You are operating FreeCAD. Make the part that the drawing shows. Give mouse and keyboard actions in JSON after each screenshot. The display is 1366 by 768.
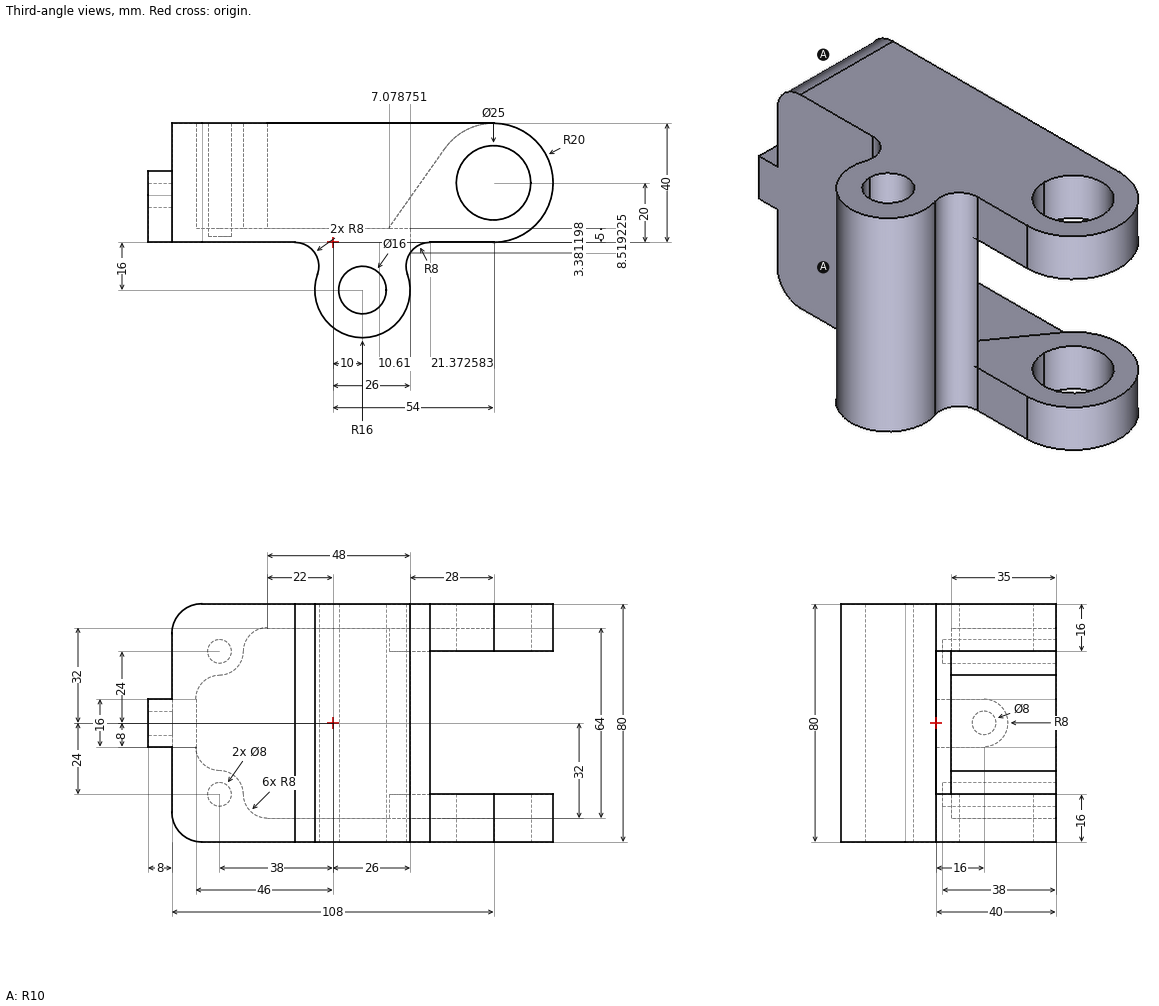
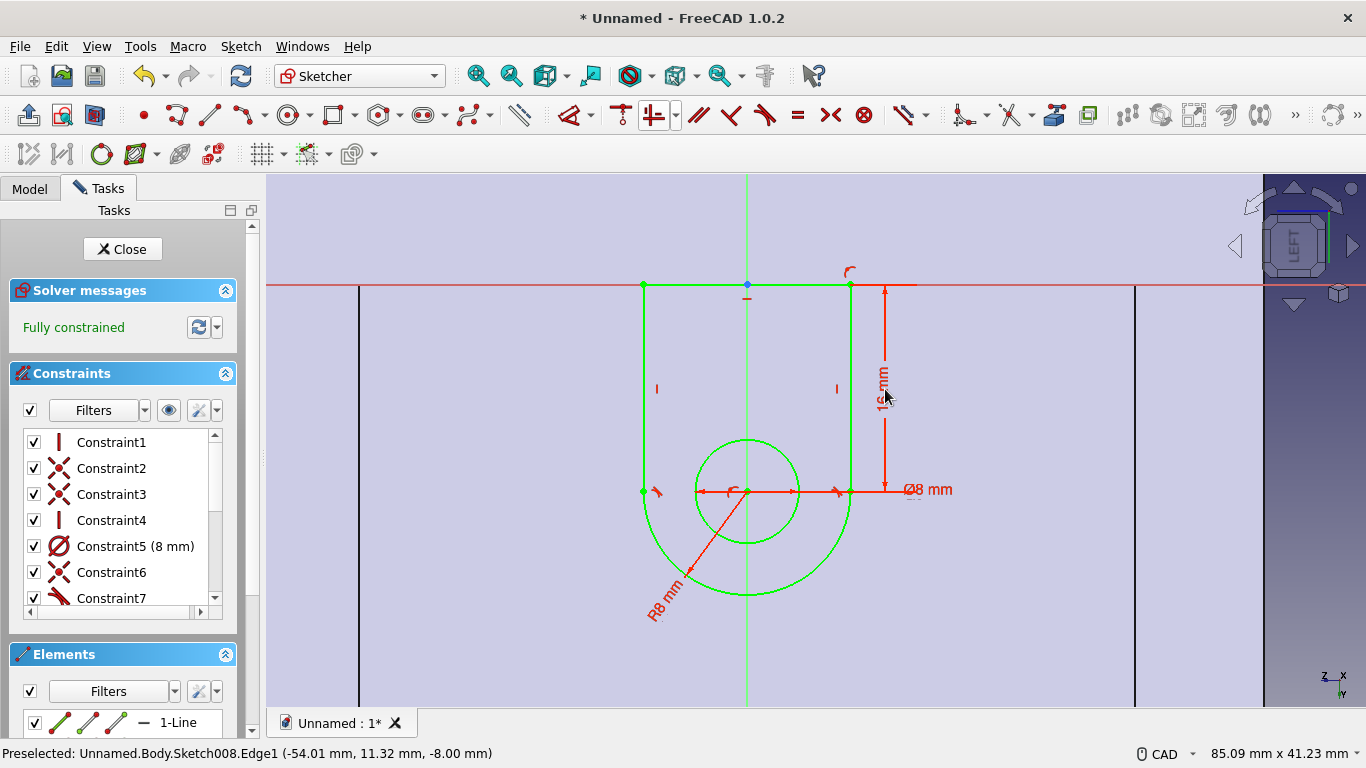
{"action": "left_click", "coordinate": [123, 249]}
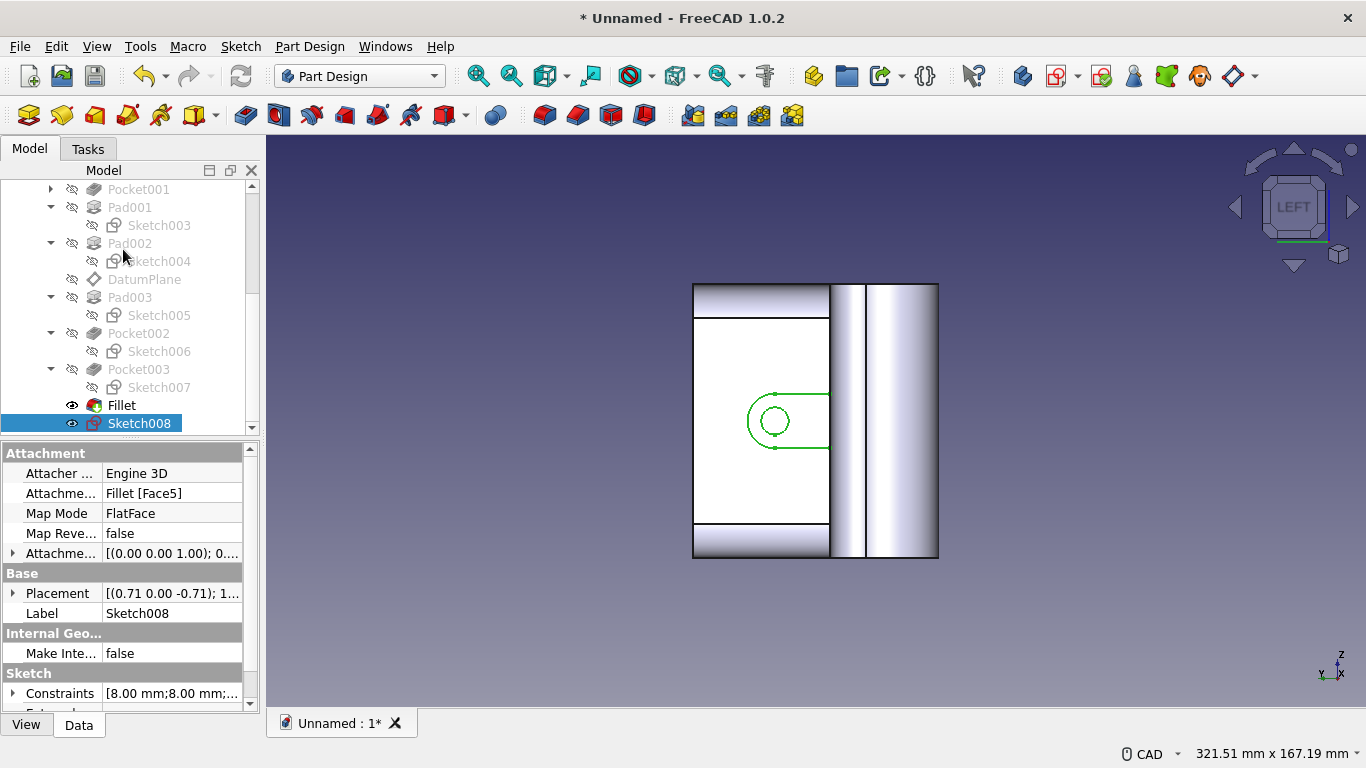
{"action": "left_click", "coordinate": [29, 116]}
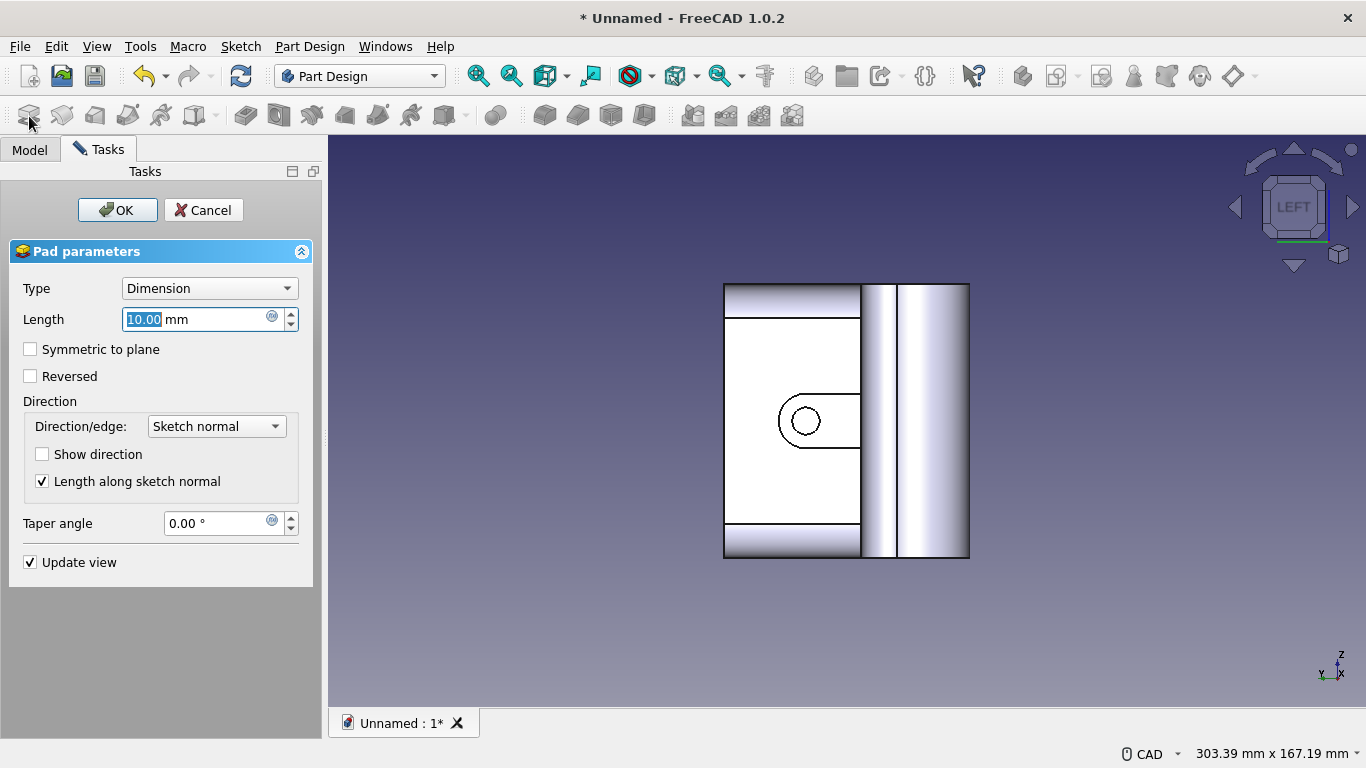
{"action": "type", "text": "8"}
{"action": "key", "text": "Tab"}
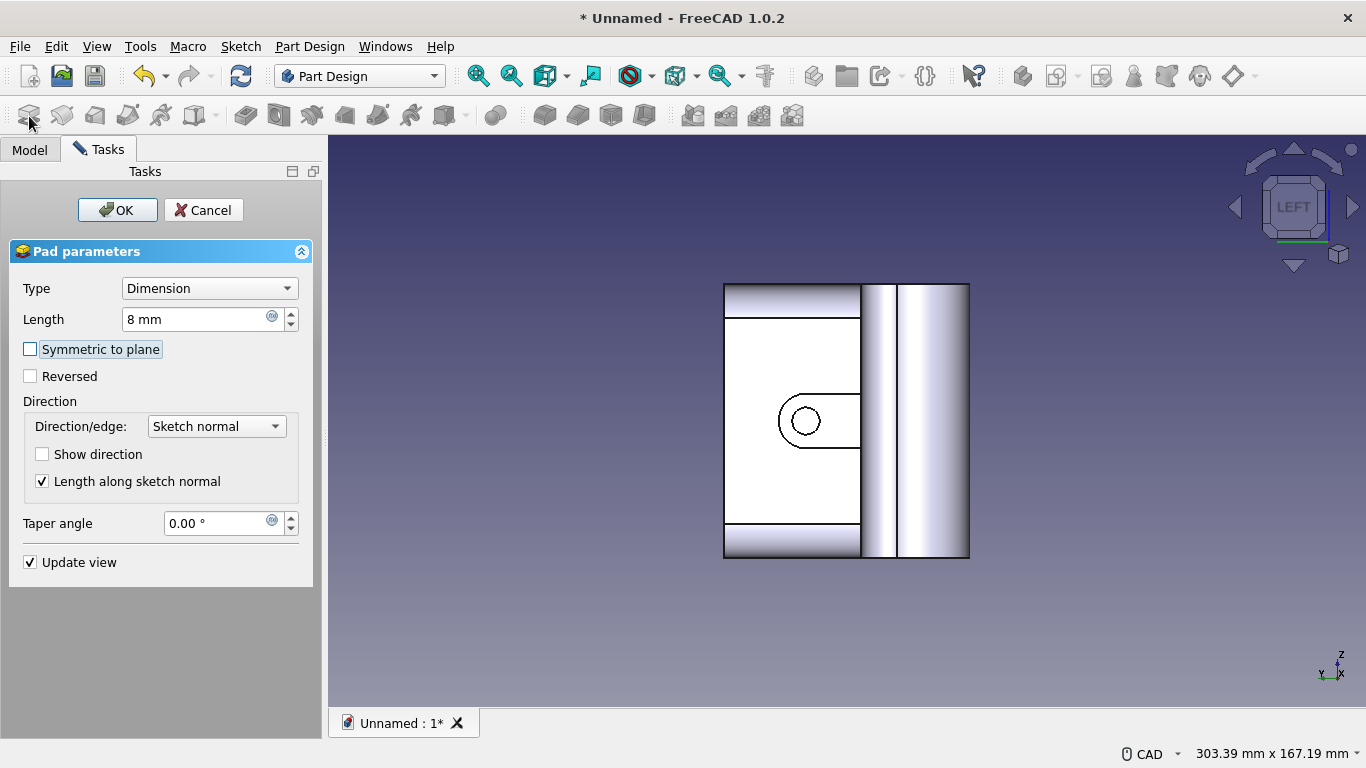
{"action": "left_click", "coordinate": [118, 210]}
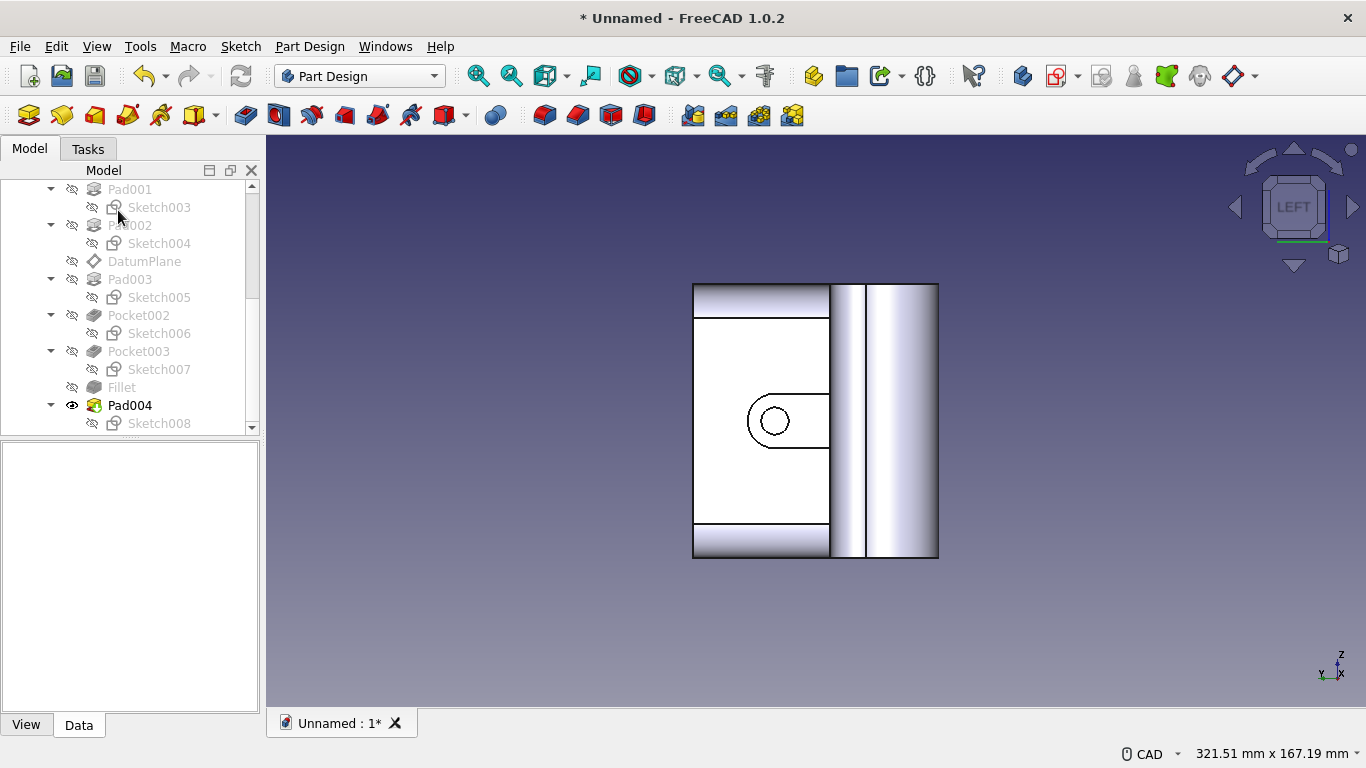
{"action": "key", "text": "0"}